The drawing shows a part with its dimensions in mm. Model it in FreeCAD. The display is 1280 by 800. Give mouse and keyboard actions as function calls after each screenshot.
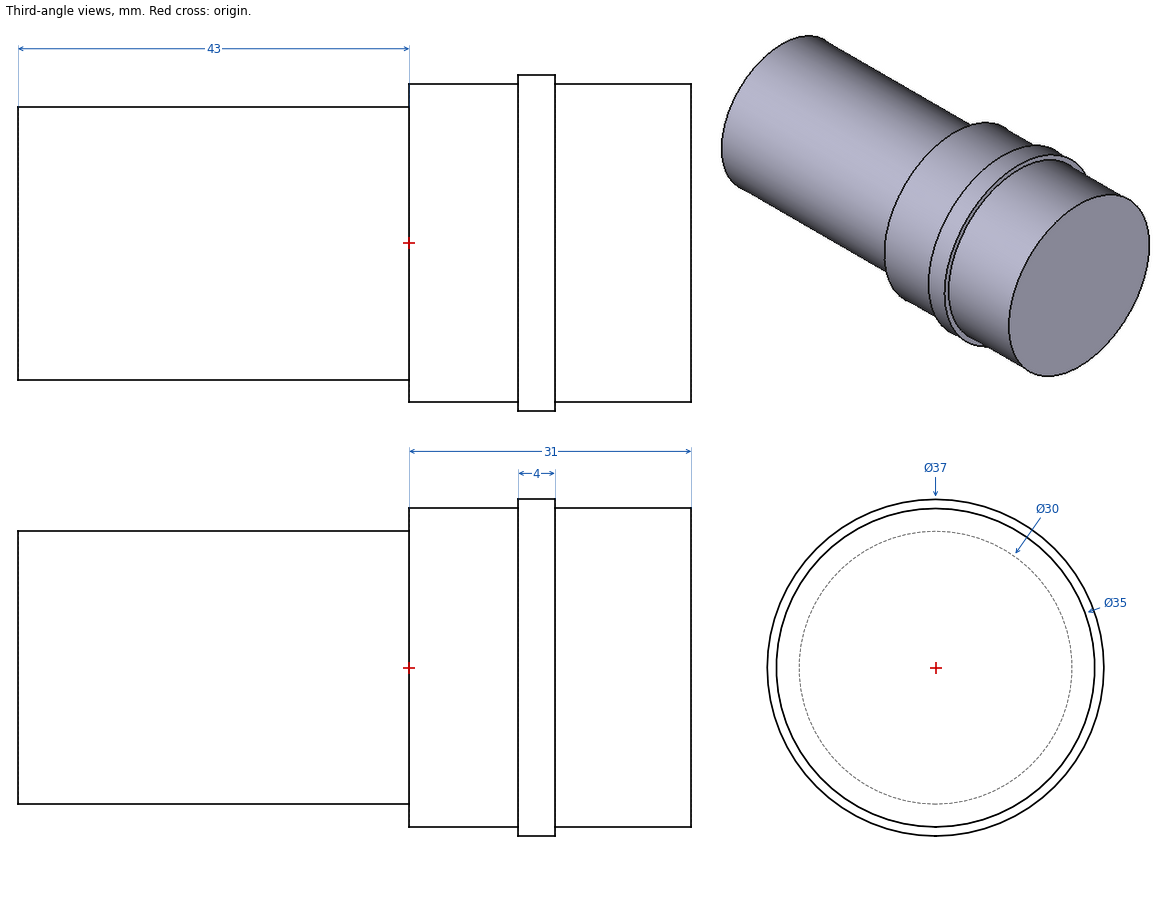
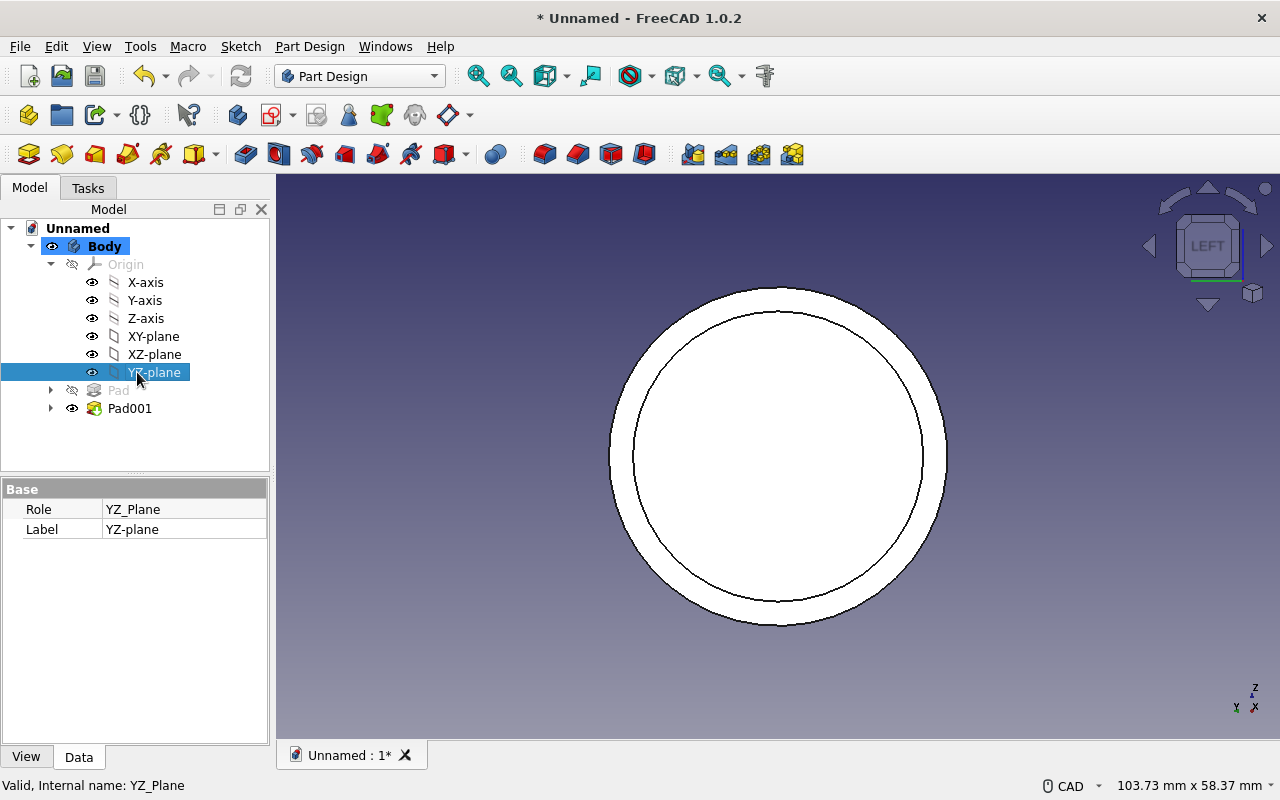
click(448, 116)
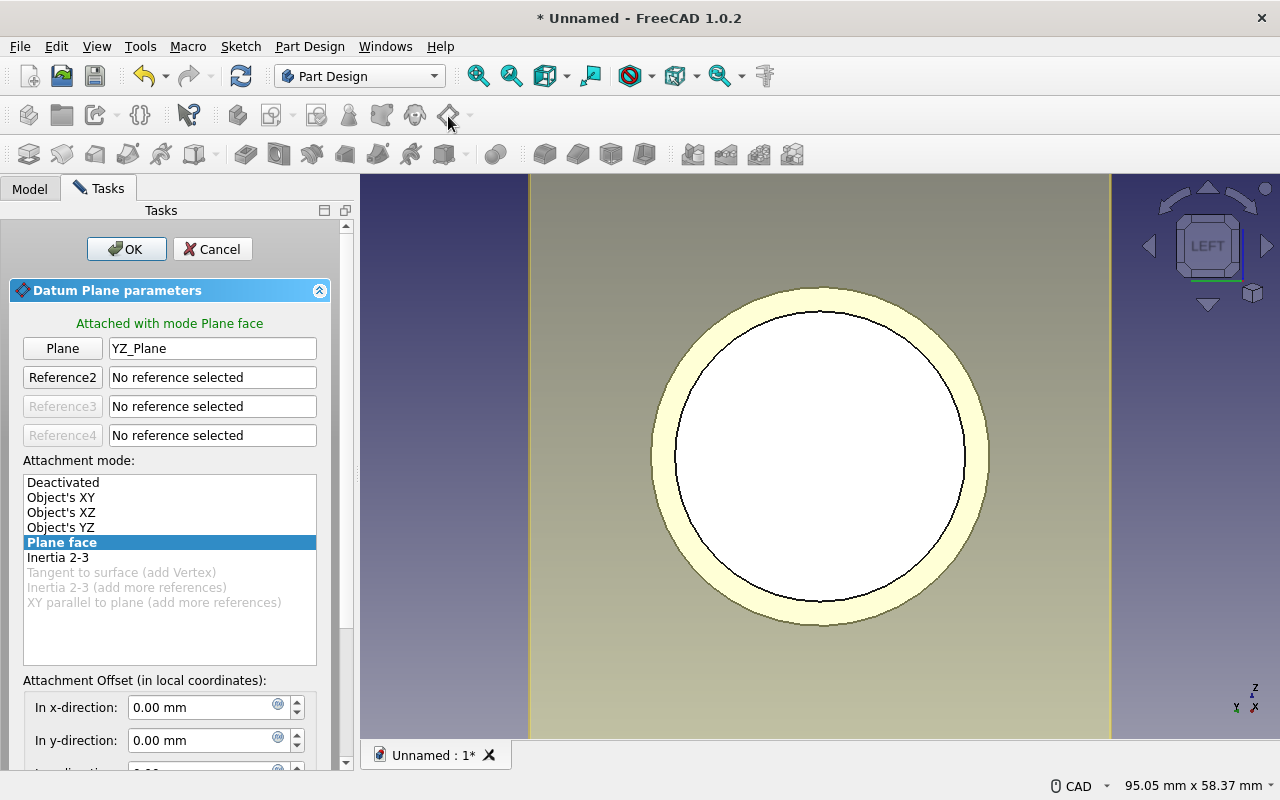
scroll(346, 495, down, 2)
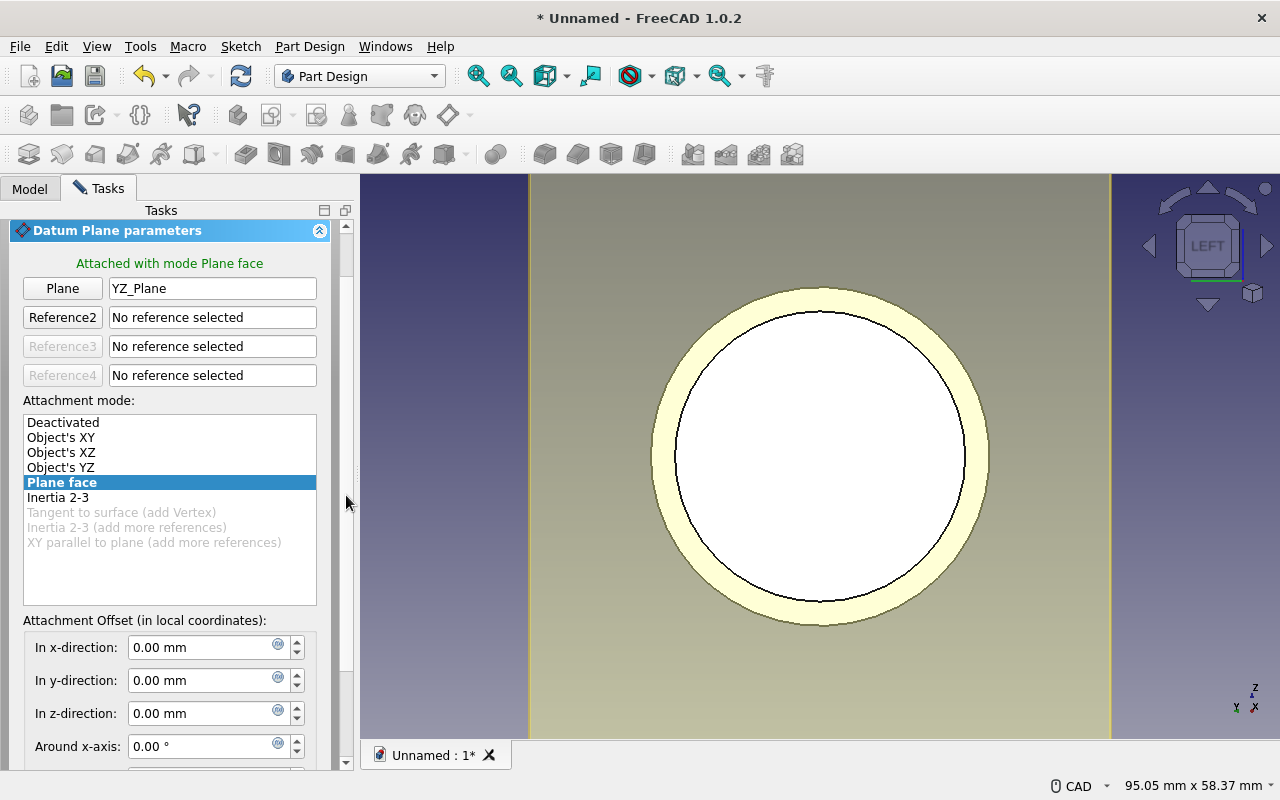
triple_click(210, 654)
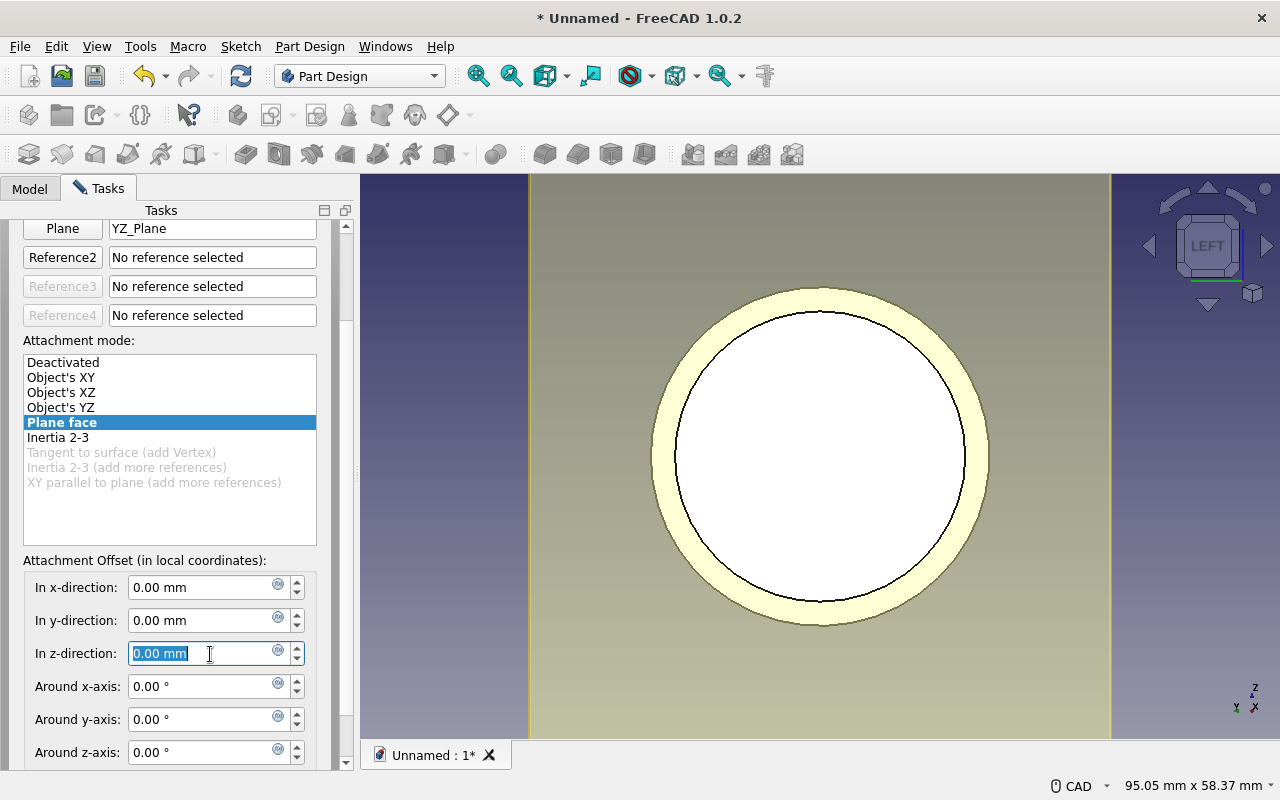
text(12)
key(Tab)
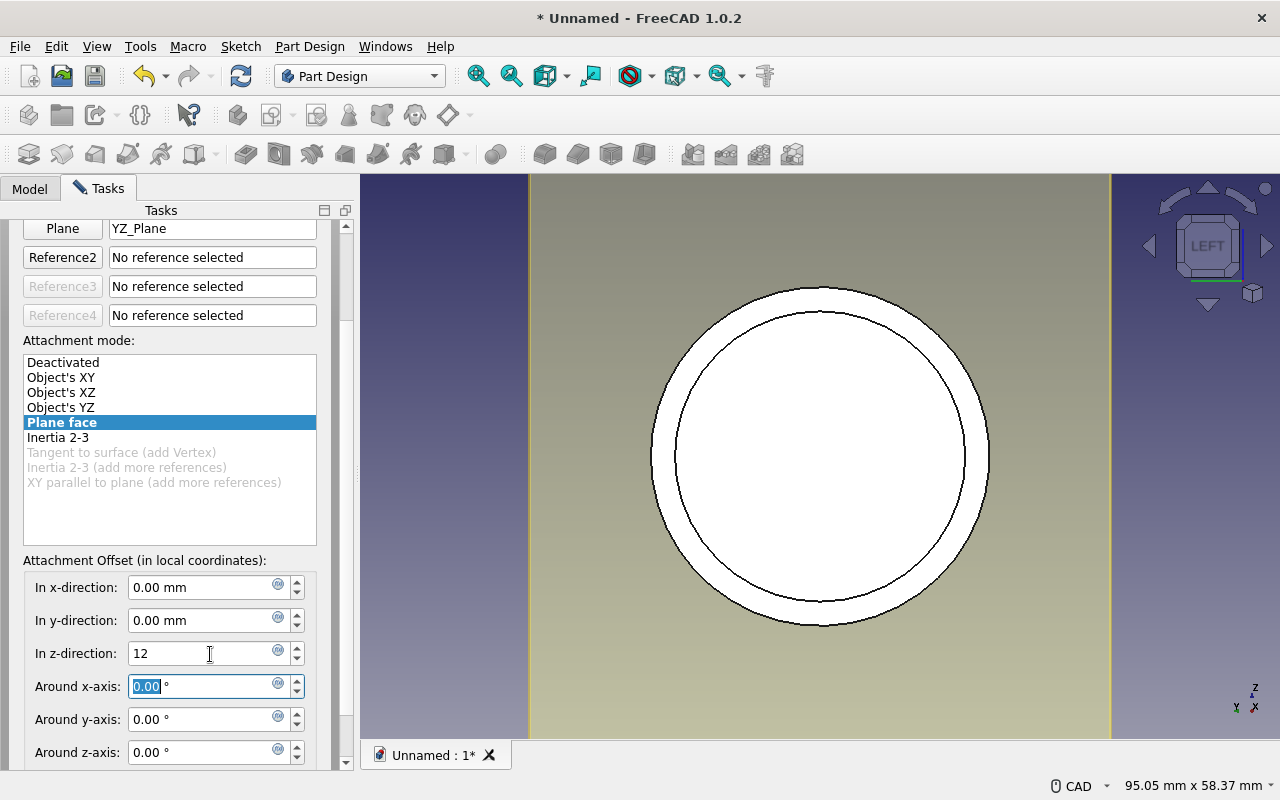
scroll(346, 495, up, 3)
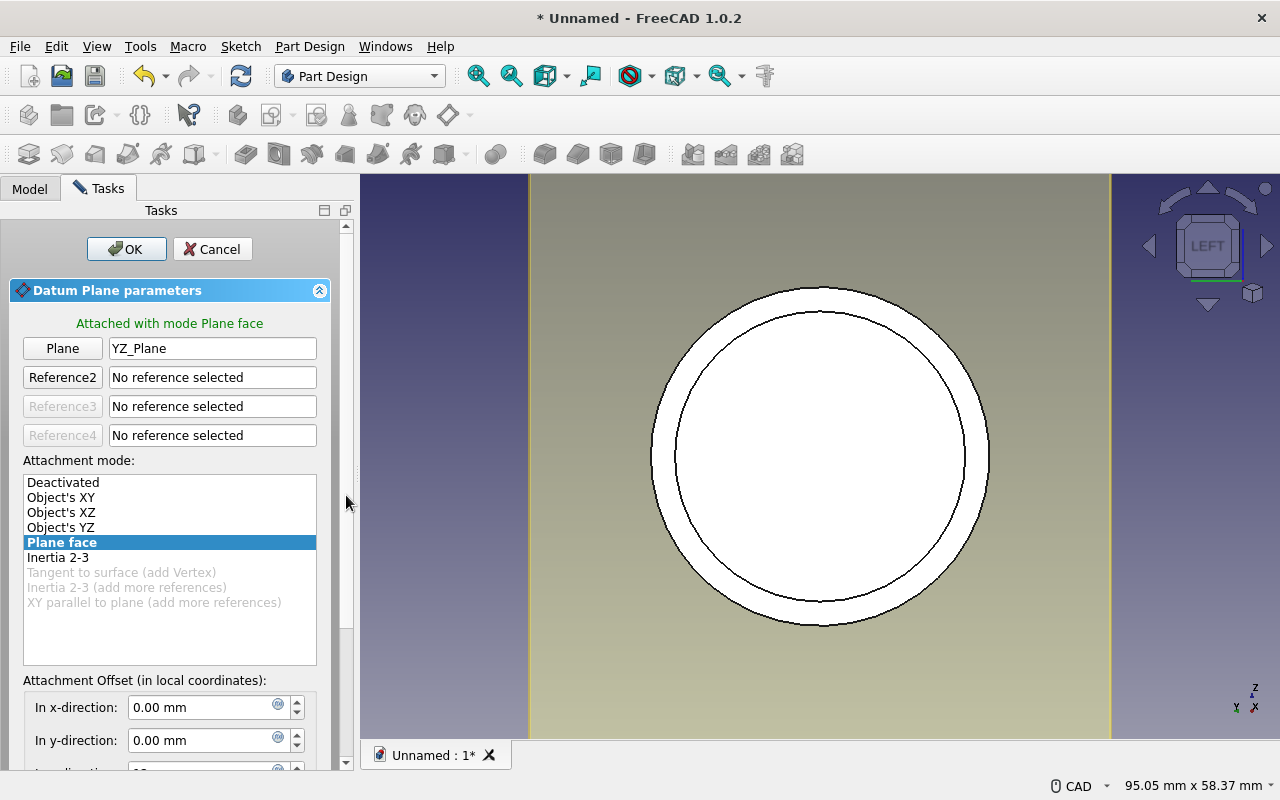
click(127, 249)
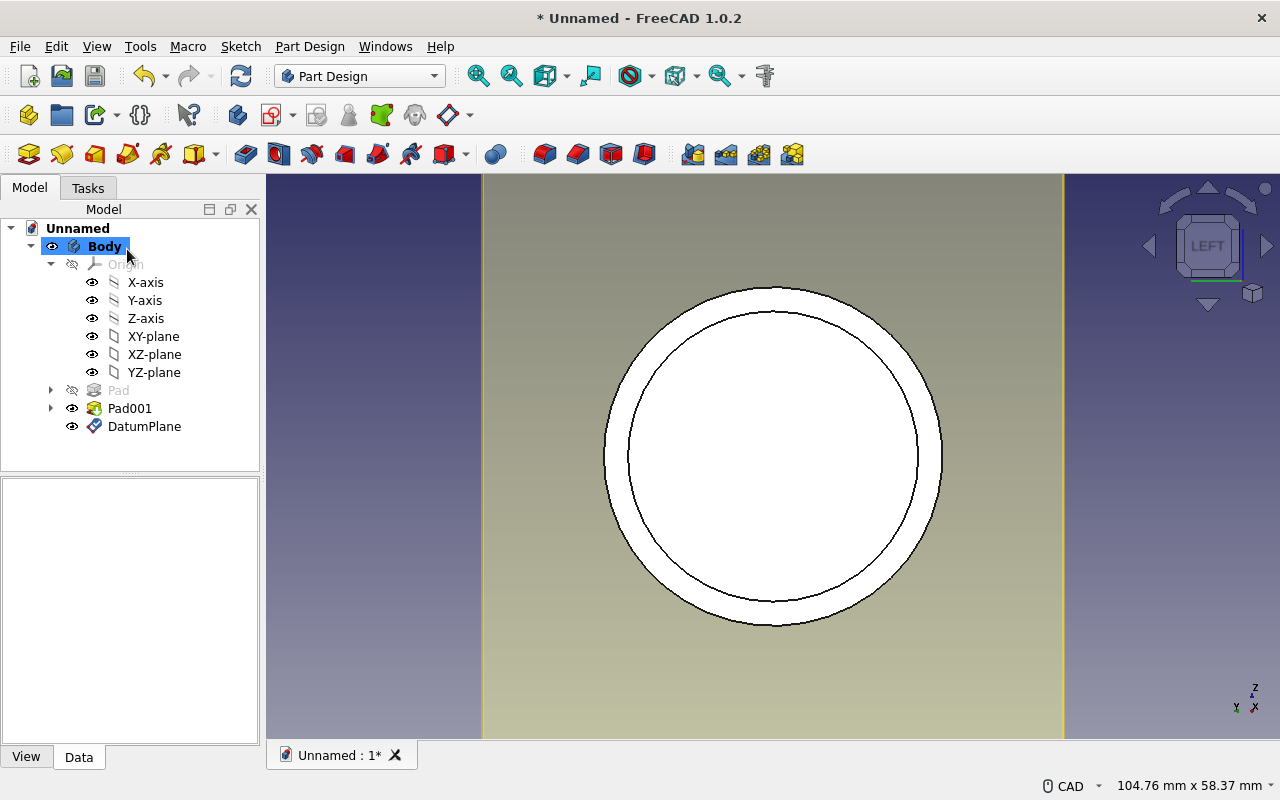
click(117, 426)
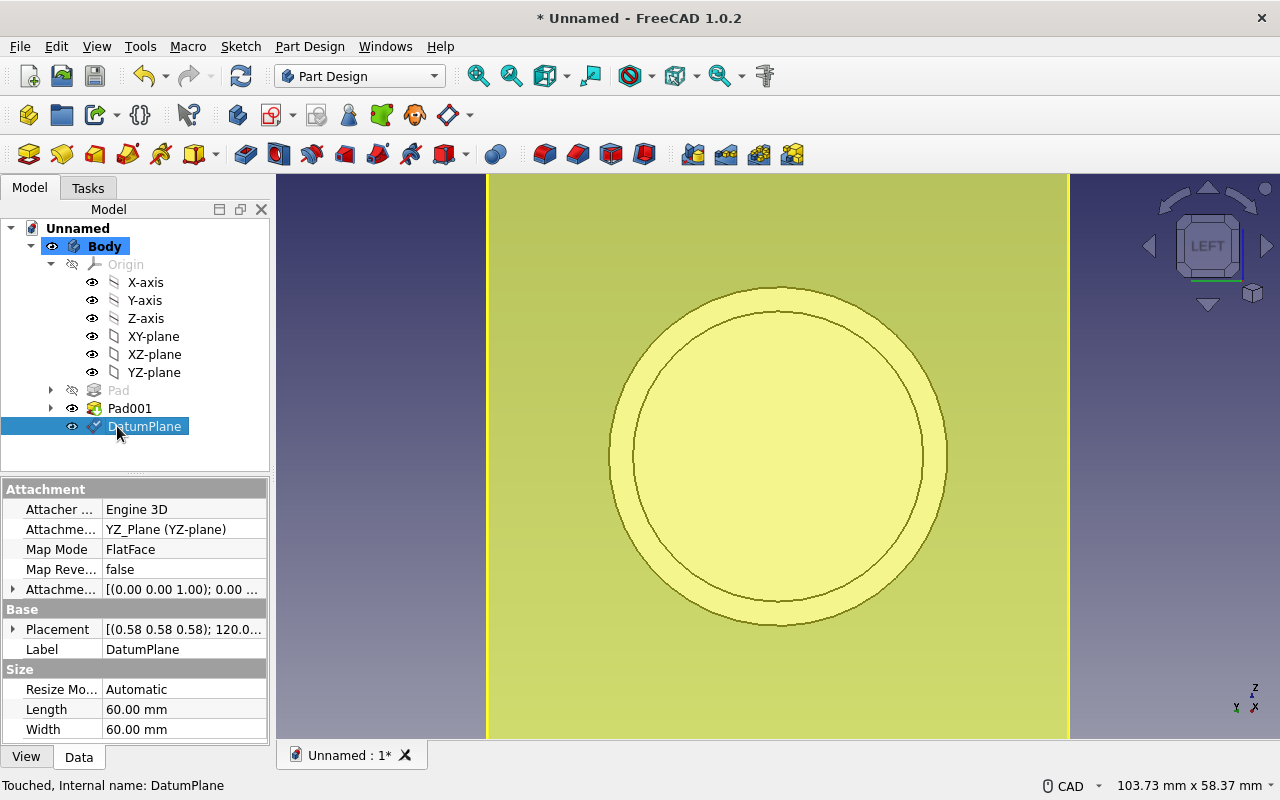
click(270, 116)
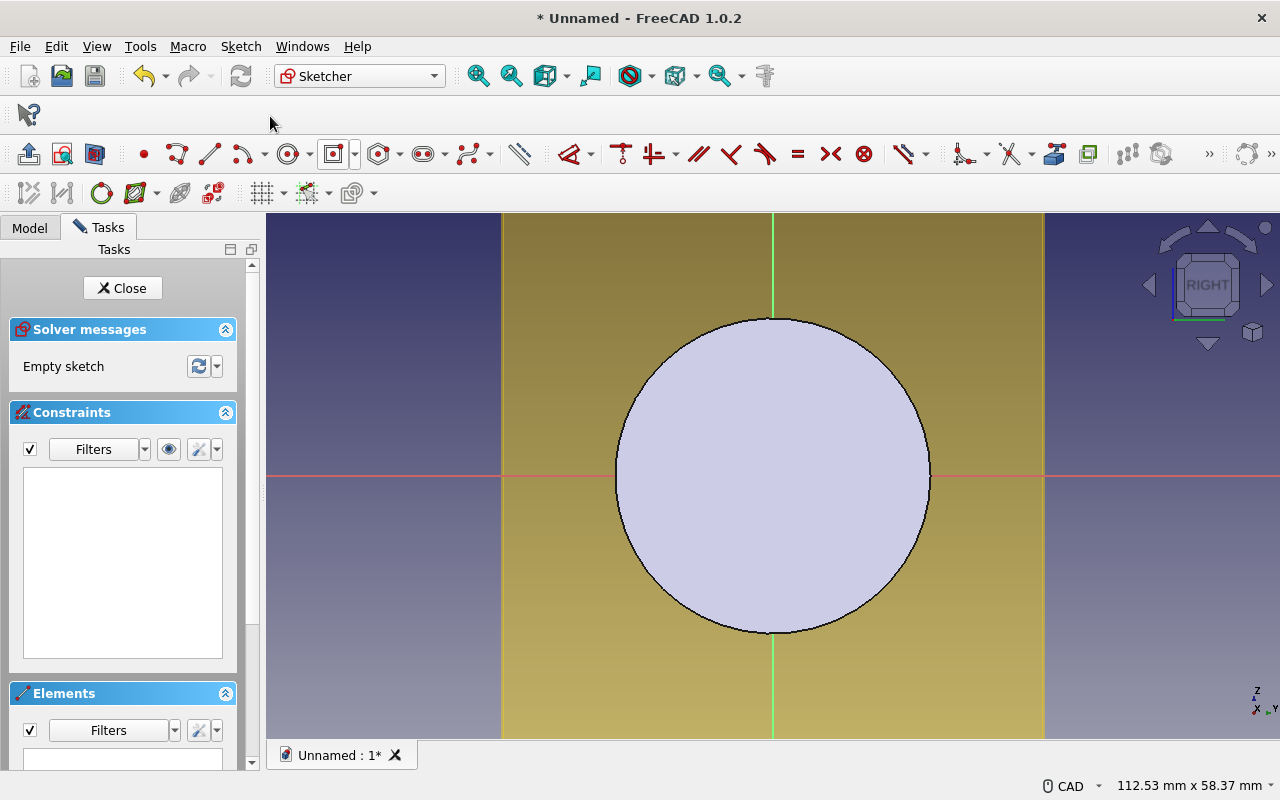
click(95, 154)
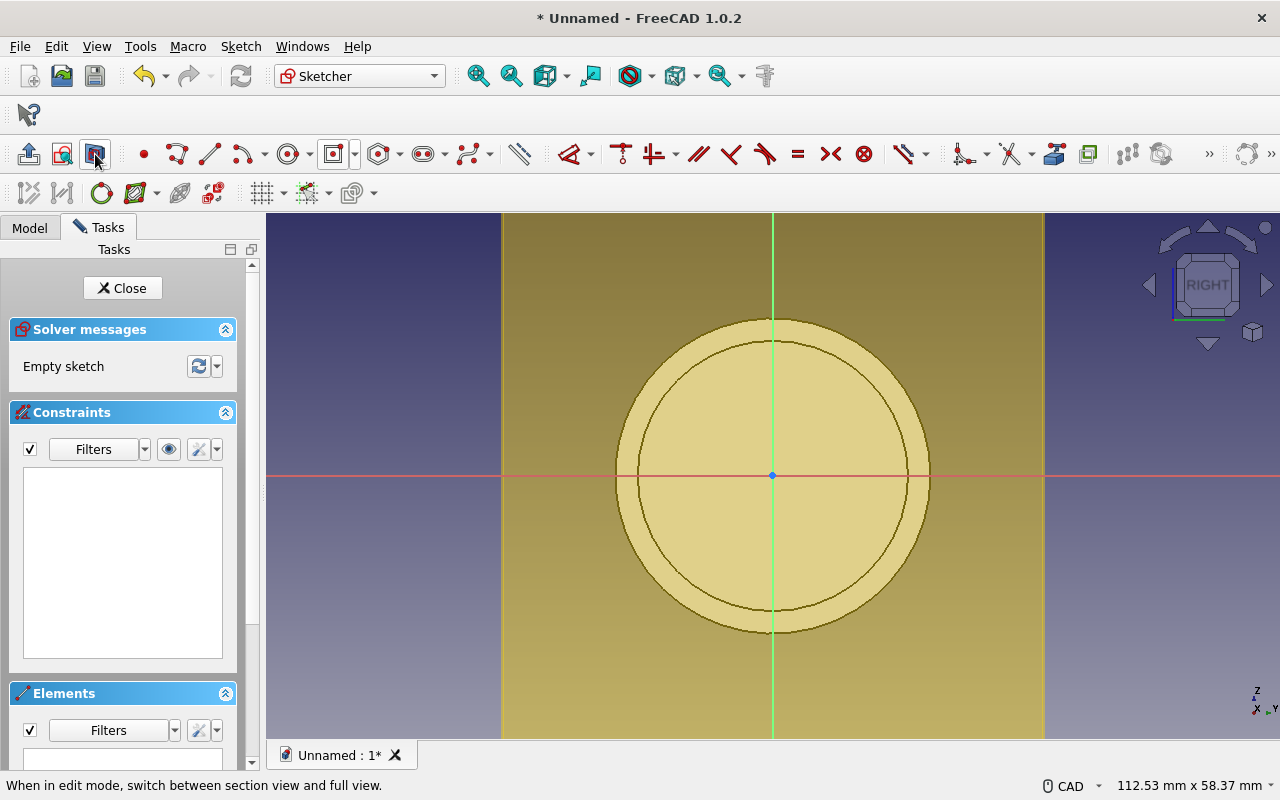
key(g)
key(c)